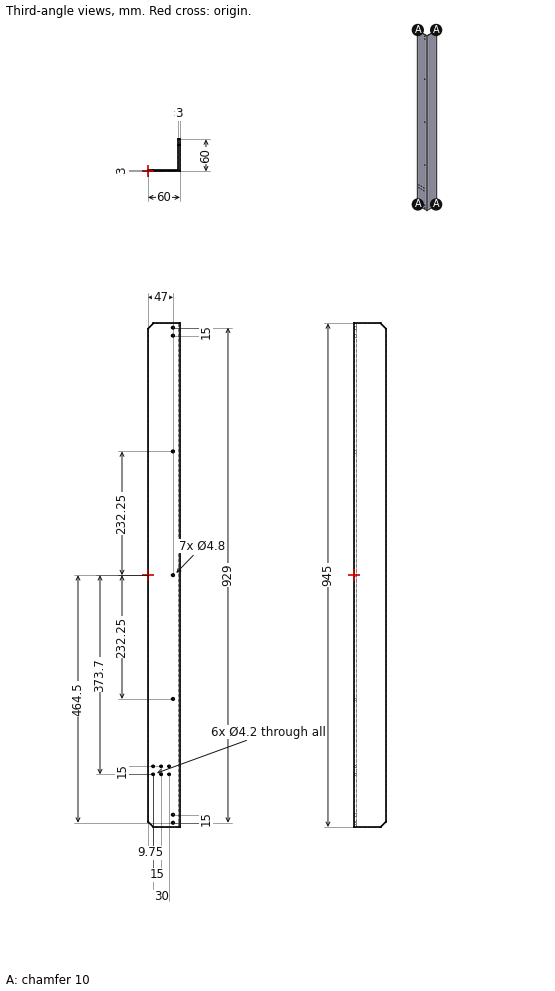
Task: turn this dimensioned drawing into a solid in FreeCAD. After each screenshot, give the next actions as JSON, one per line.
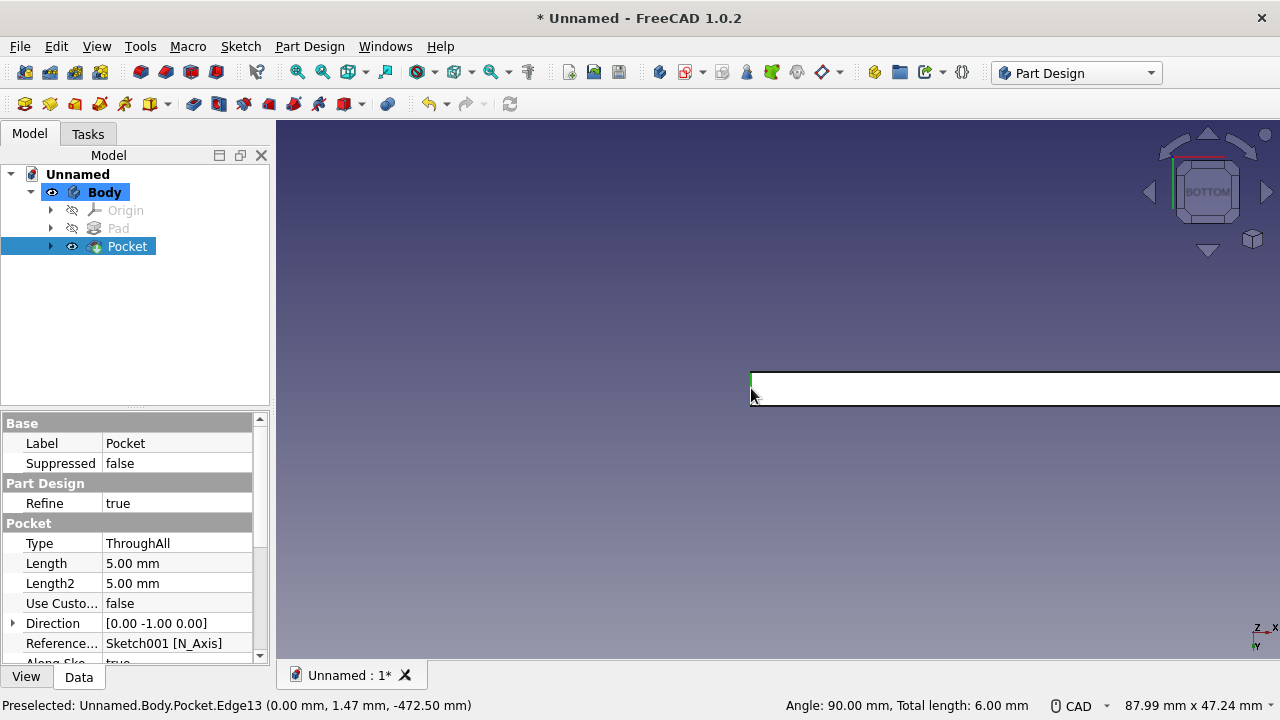
{"action": "left_click", "coordinate": [298, 72]}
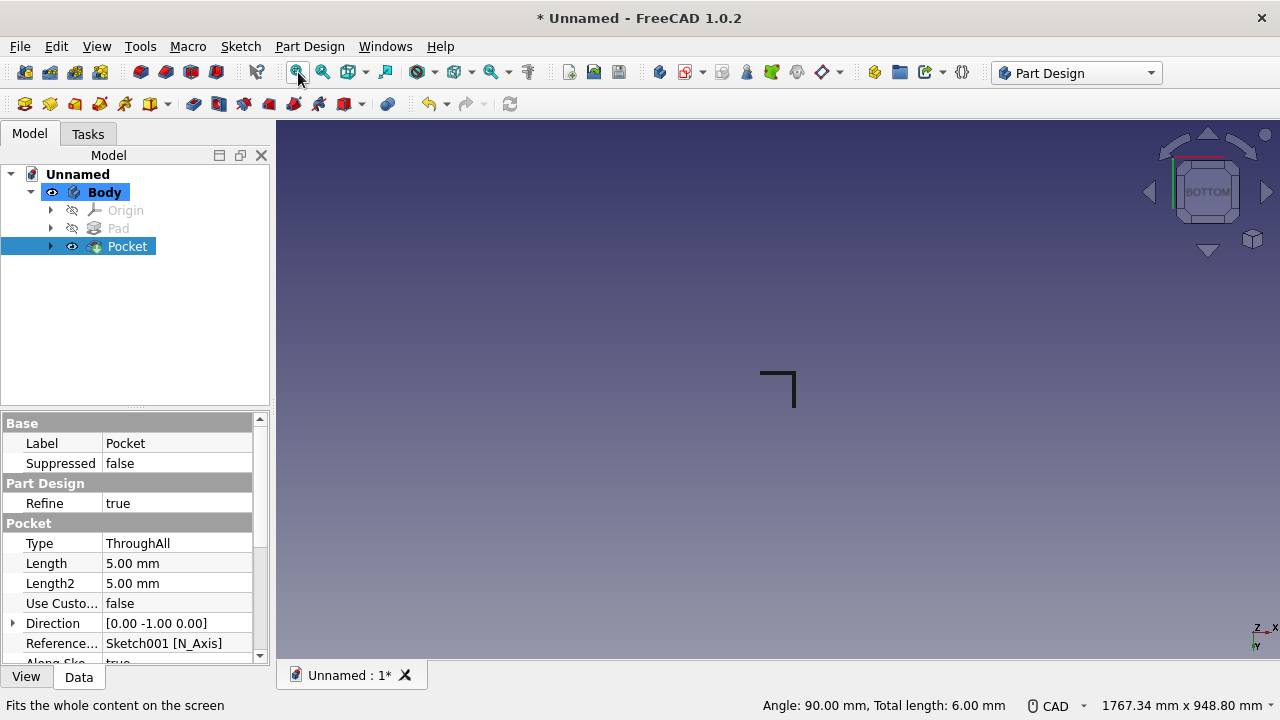
{"action": "key", "text": "4"}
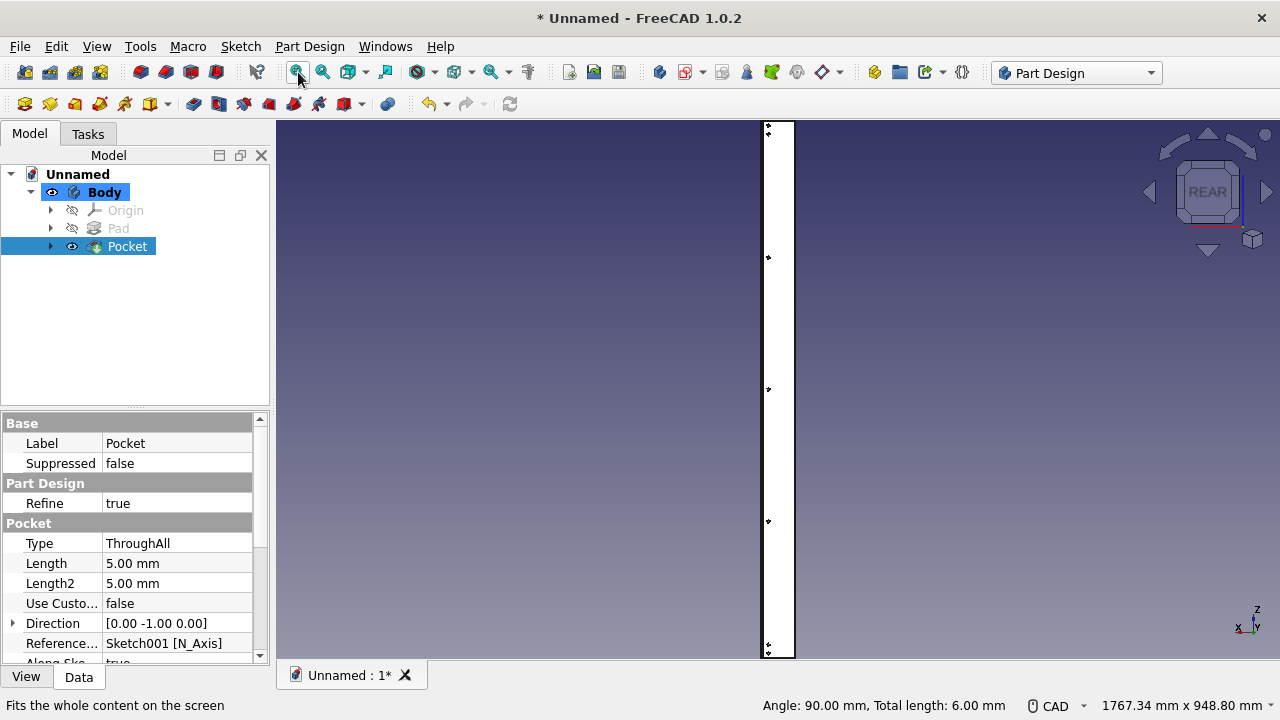
{"action": "key", "text": "6"}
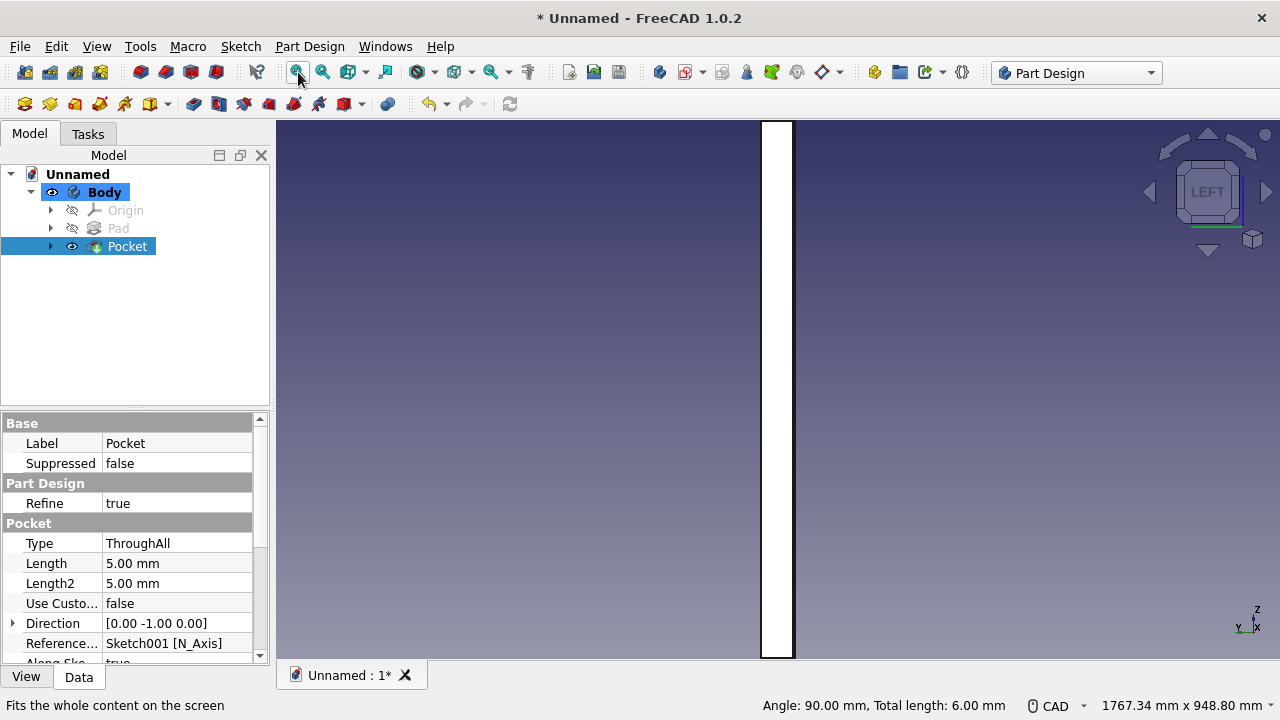
{"action": "key", "text": "v 3"}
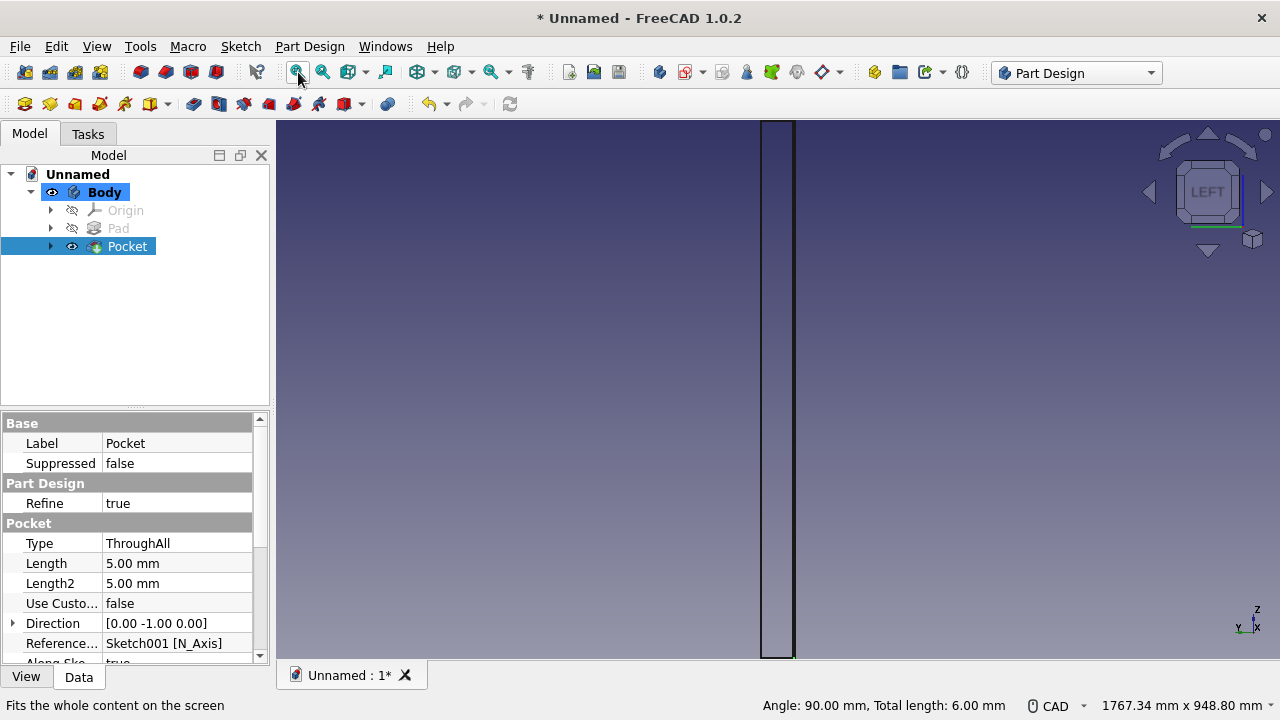
{"action": "key", "text": "0"}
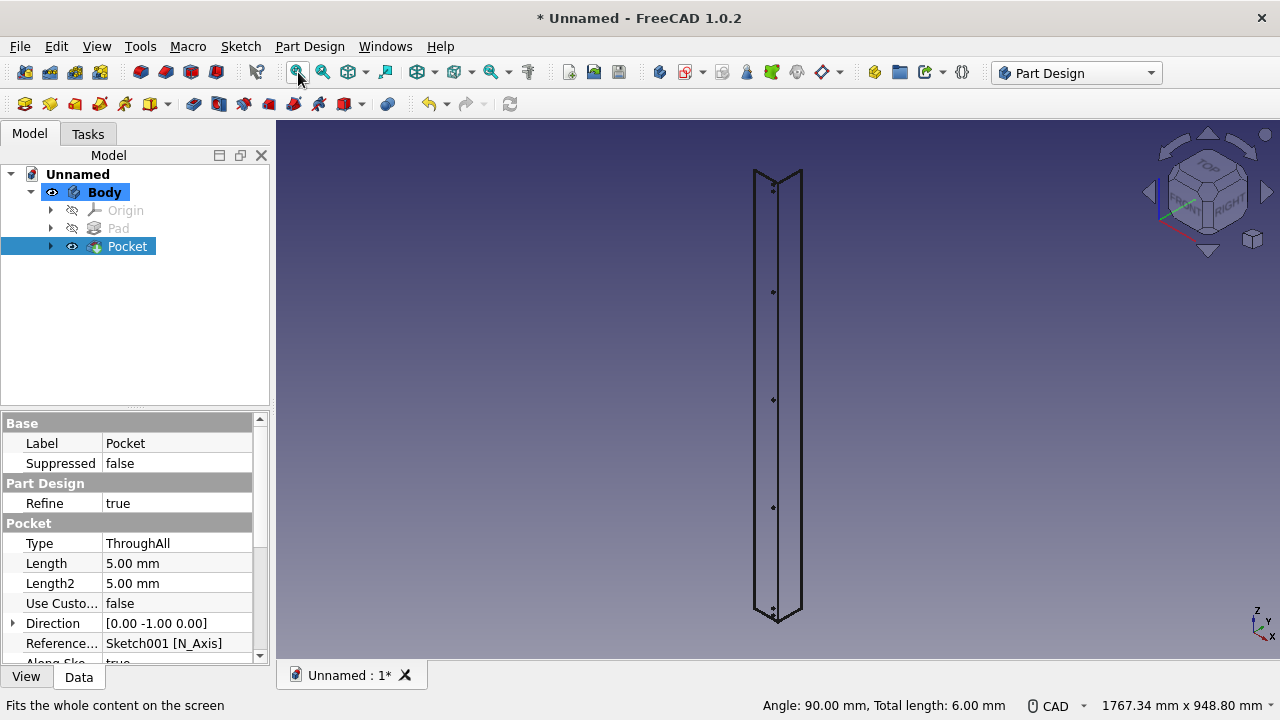
{"action": "scroll", "coordinate": [755, 169], "scroll_direction": "up", "scroll_amount": 15}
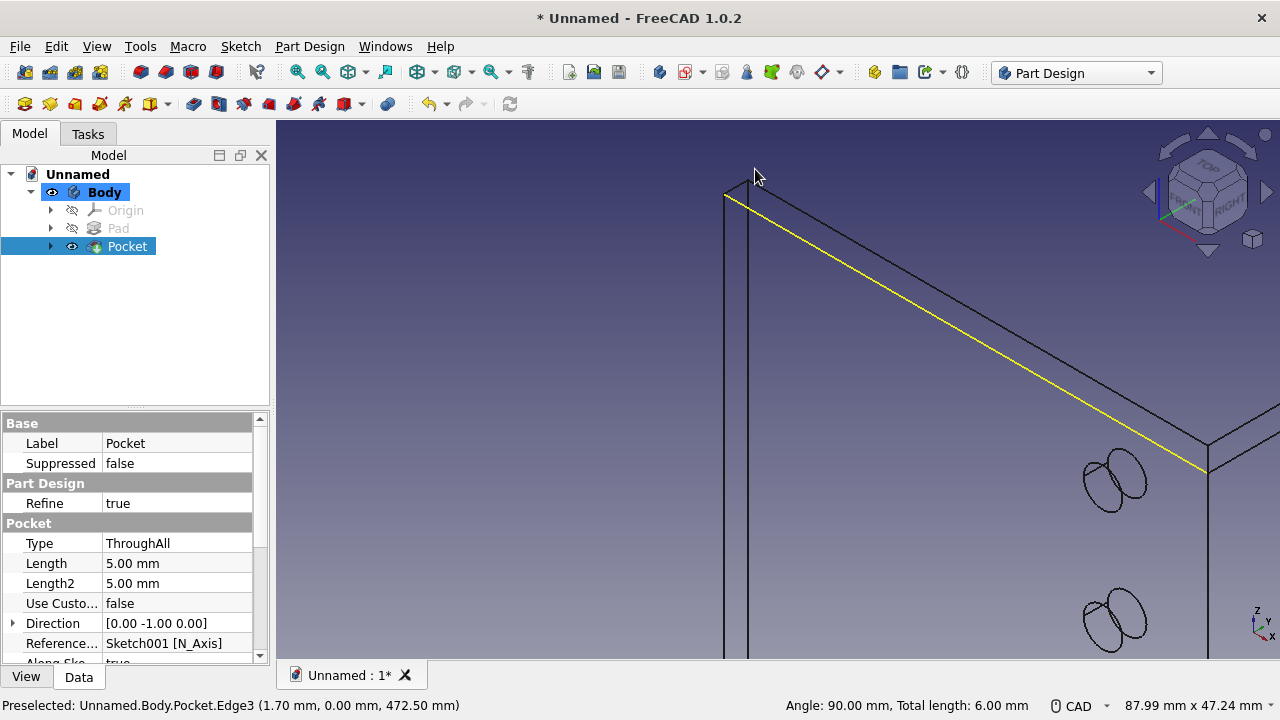
{"action": "left_click", "coordinate": [736, 186], "text": "ctrl"}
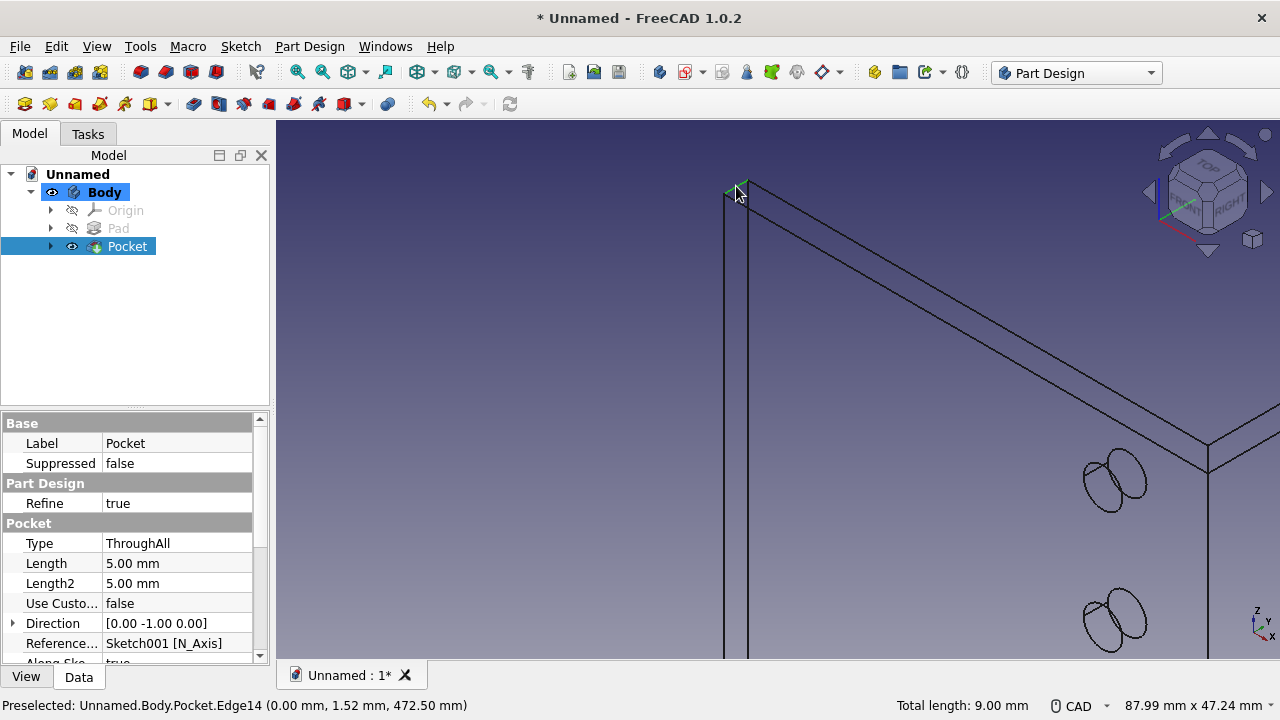
{"action": "left_click", "coordinate": [298, 72]}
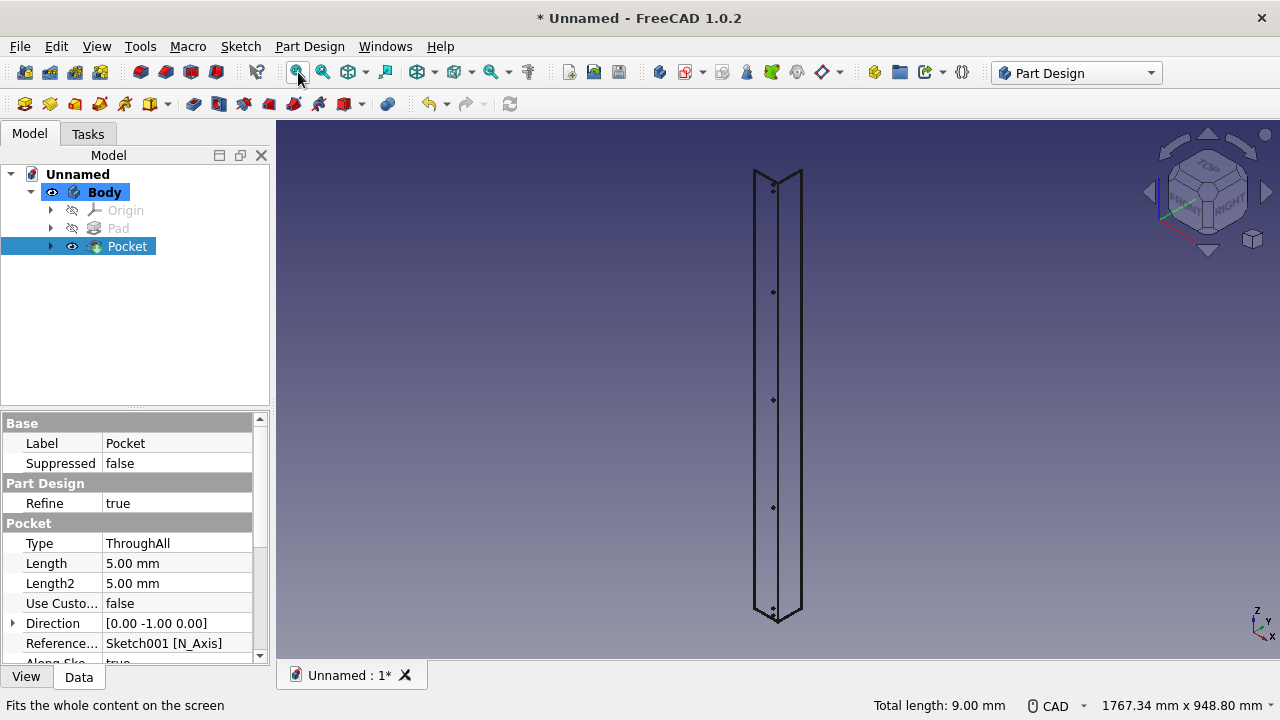
{"action": "key", "text": "2"}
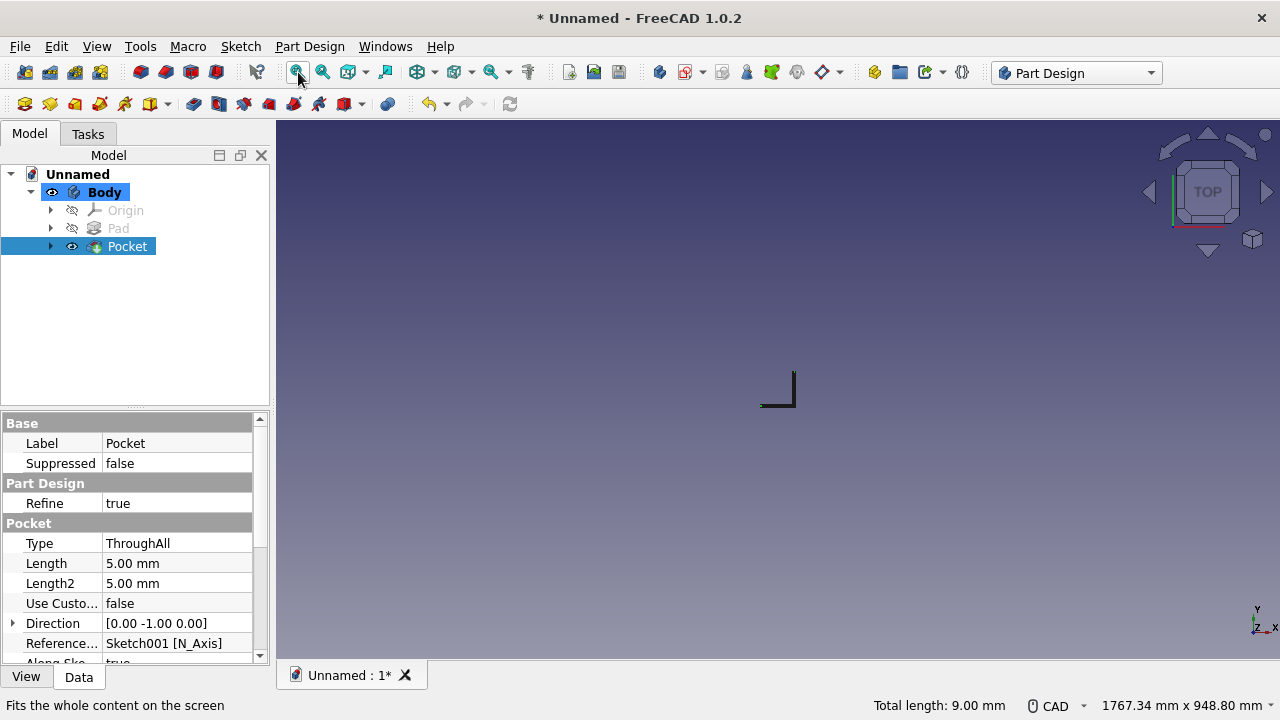
{"action": "left_click", "coordinate": [298, 72]}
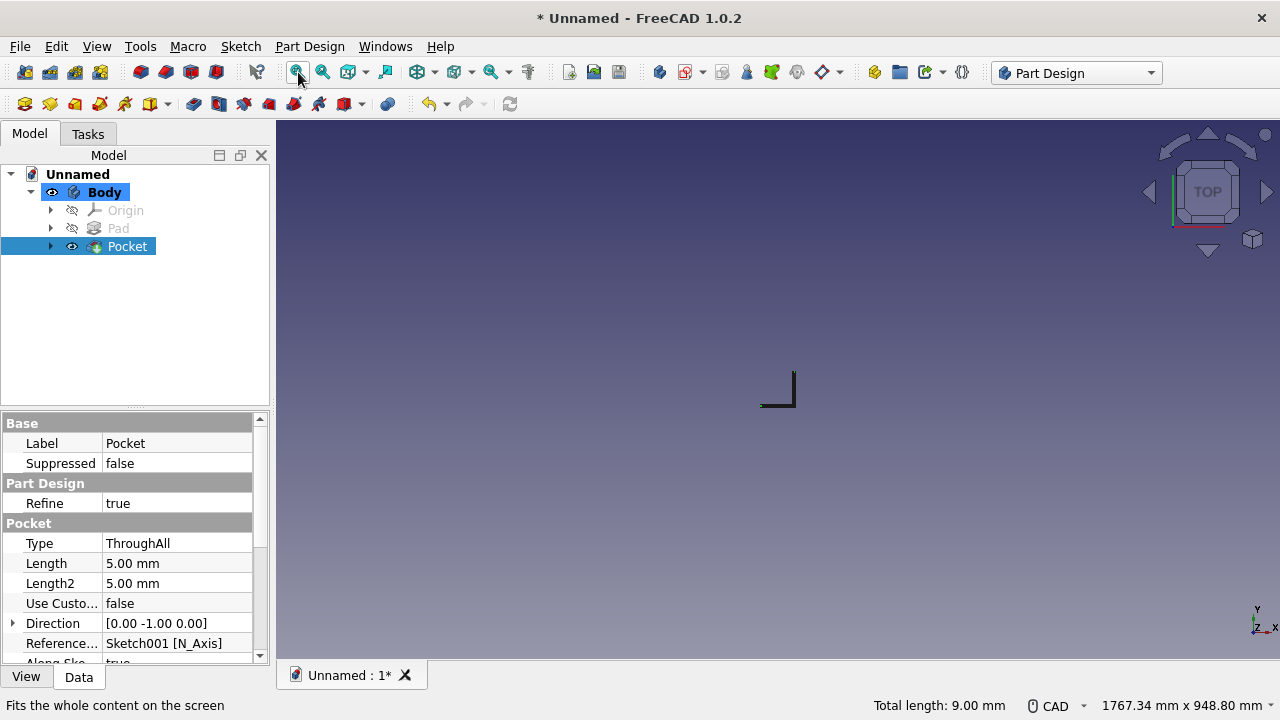
{"action": "scroll", "coordinate": [794, 371], "scroll_direction": "up", "scroll_amount": 15}